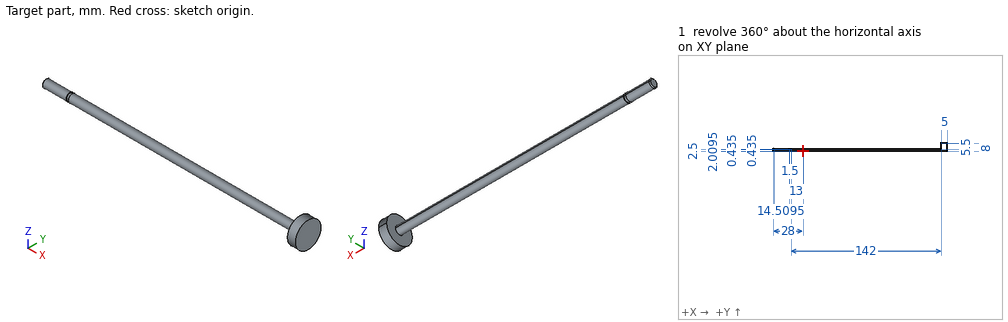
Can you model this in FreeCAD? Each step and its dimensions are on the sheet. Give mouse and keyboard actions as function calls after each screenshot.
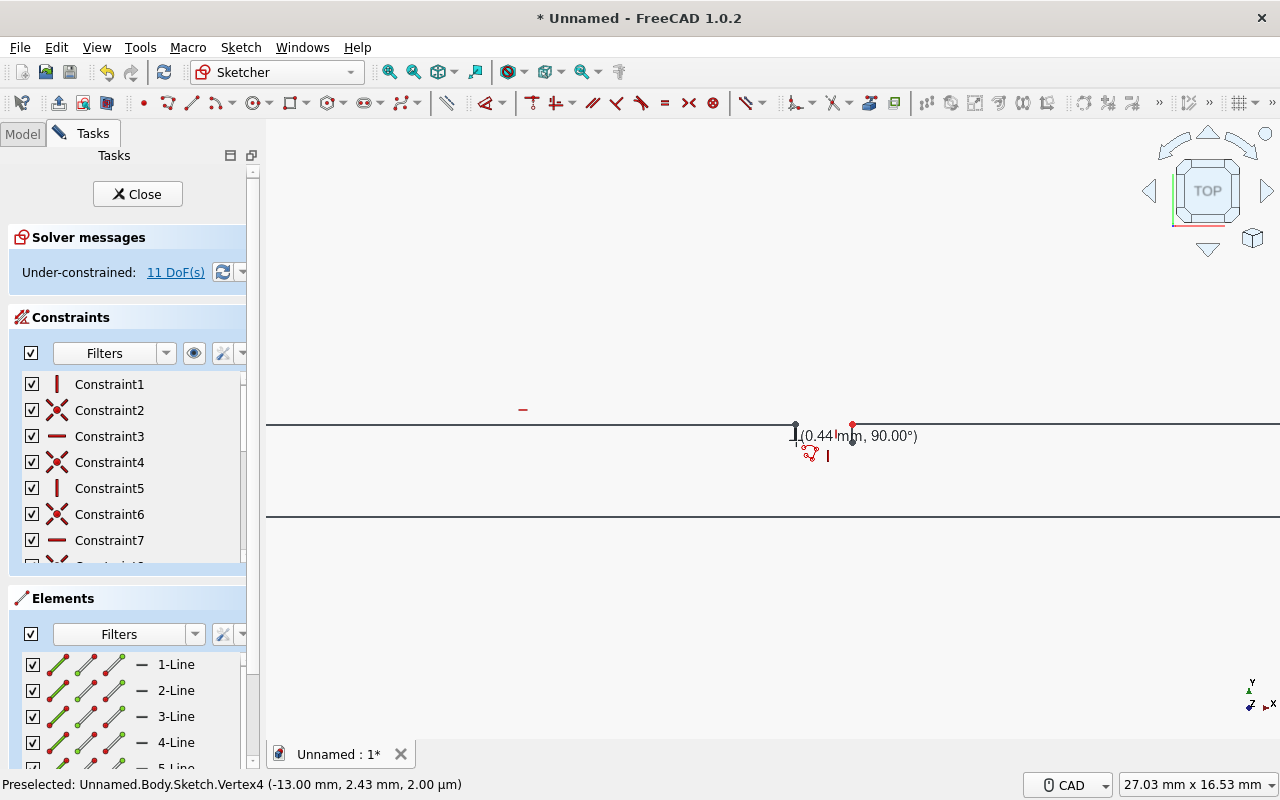
click(796, 440)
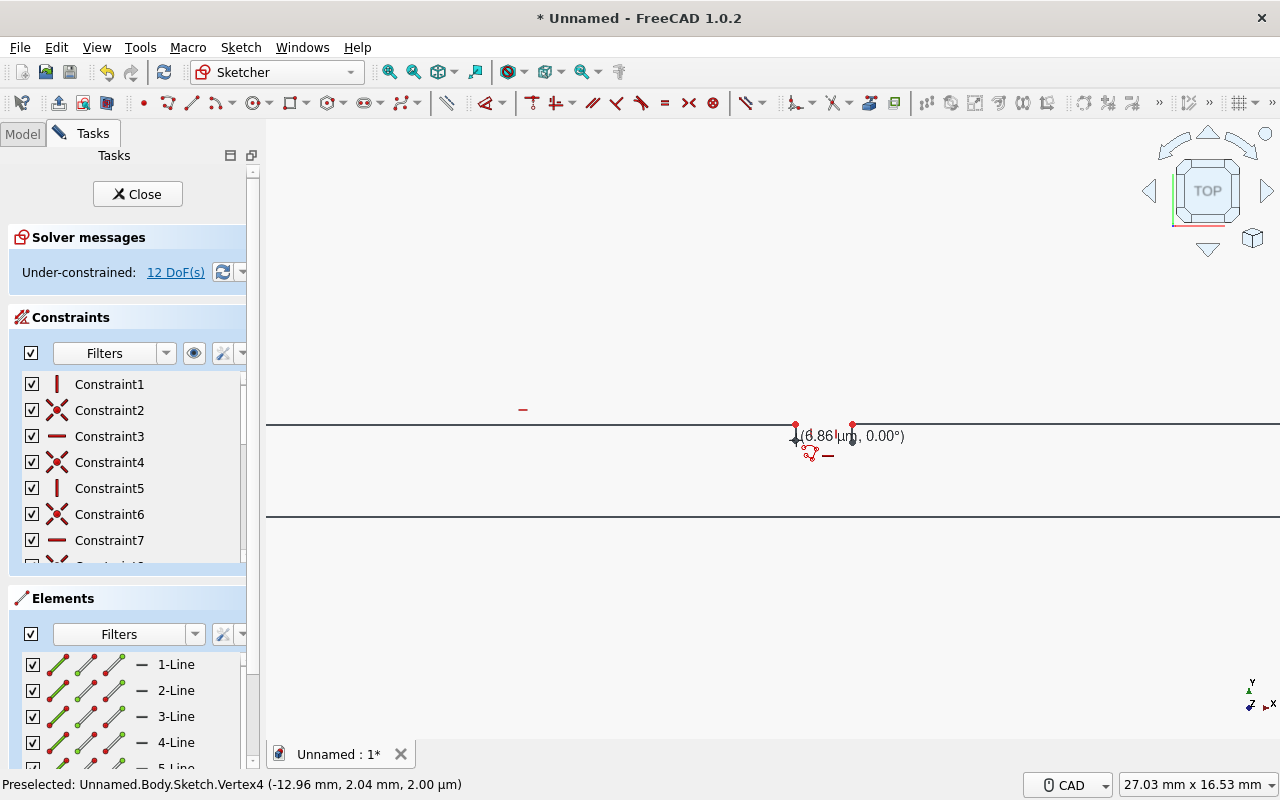
scroll(852, 440, up, 4)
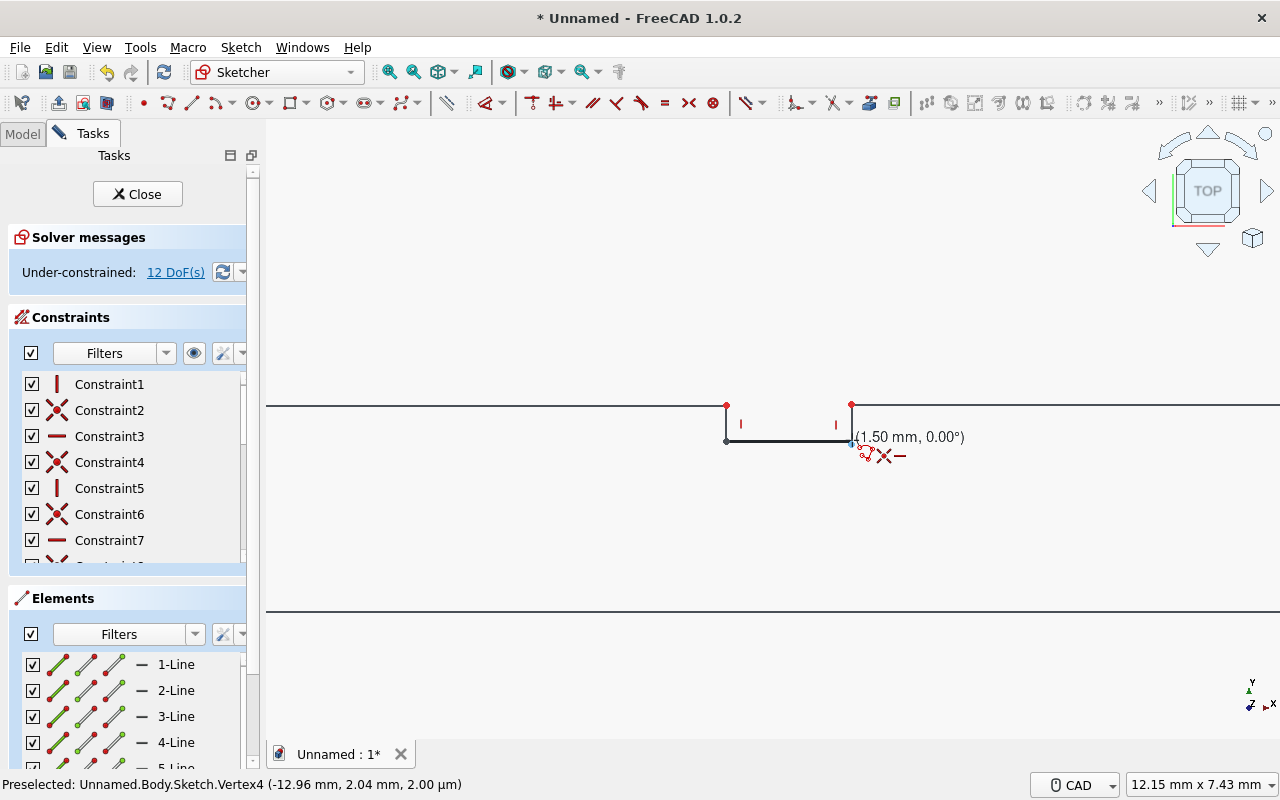
click(852, 435)
key(Escape)
key(Escape)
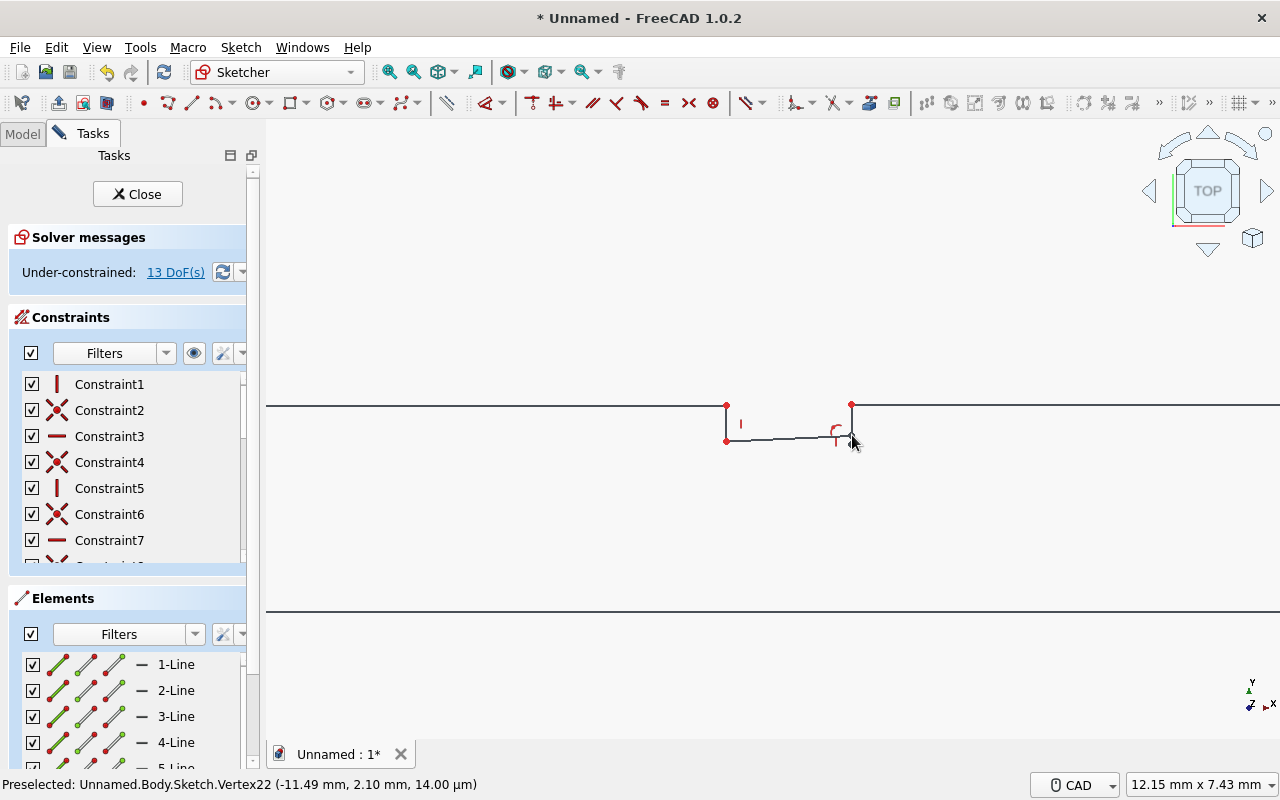
click(764, 440)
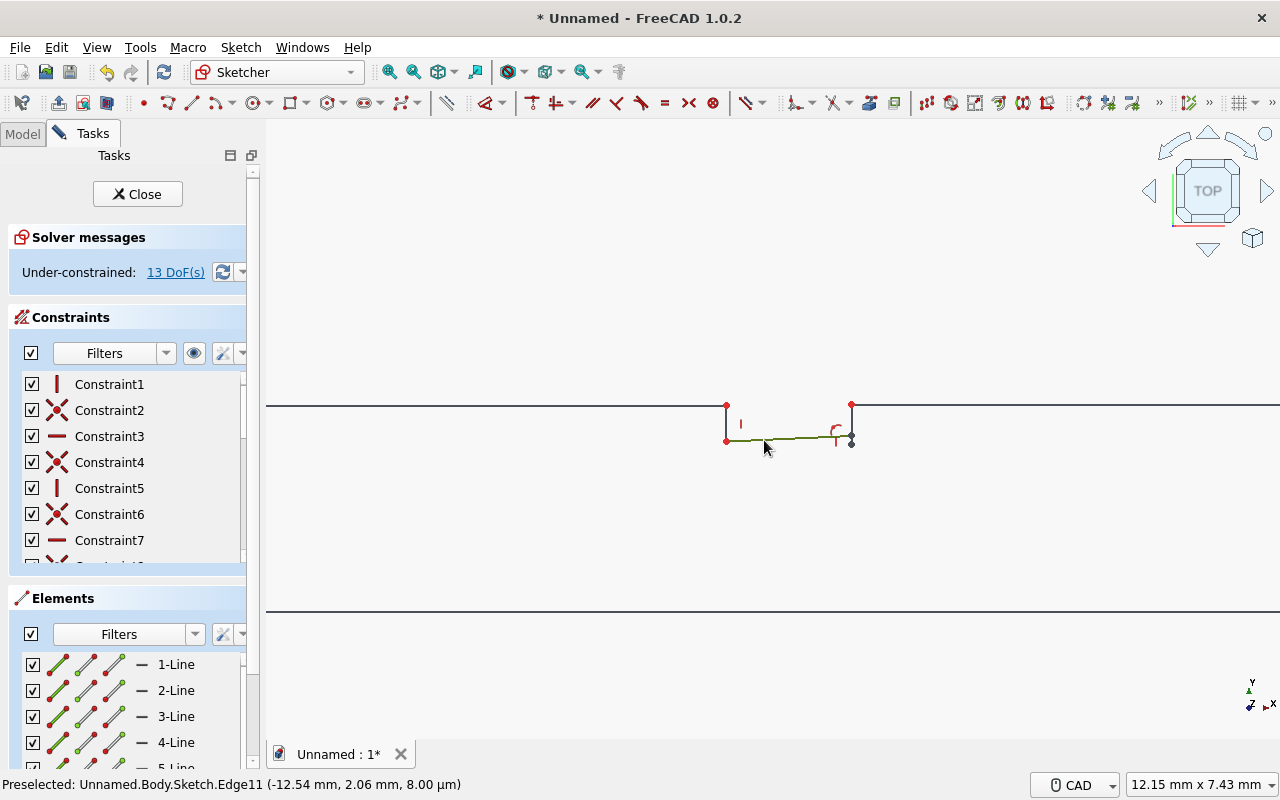
key(h)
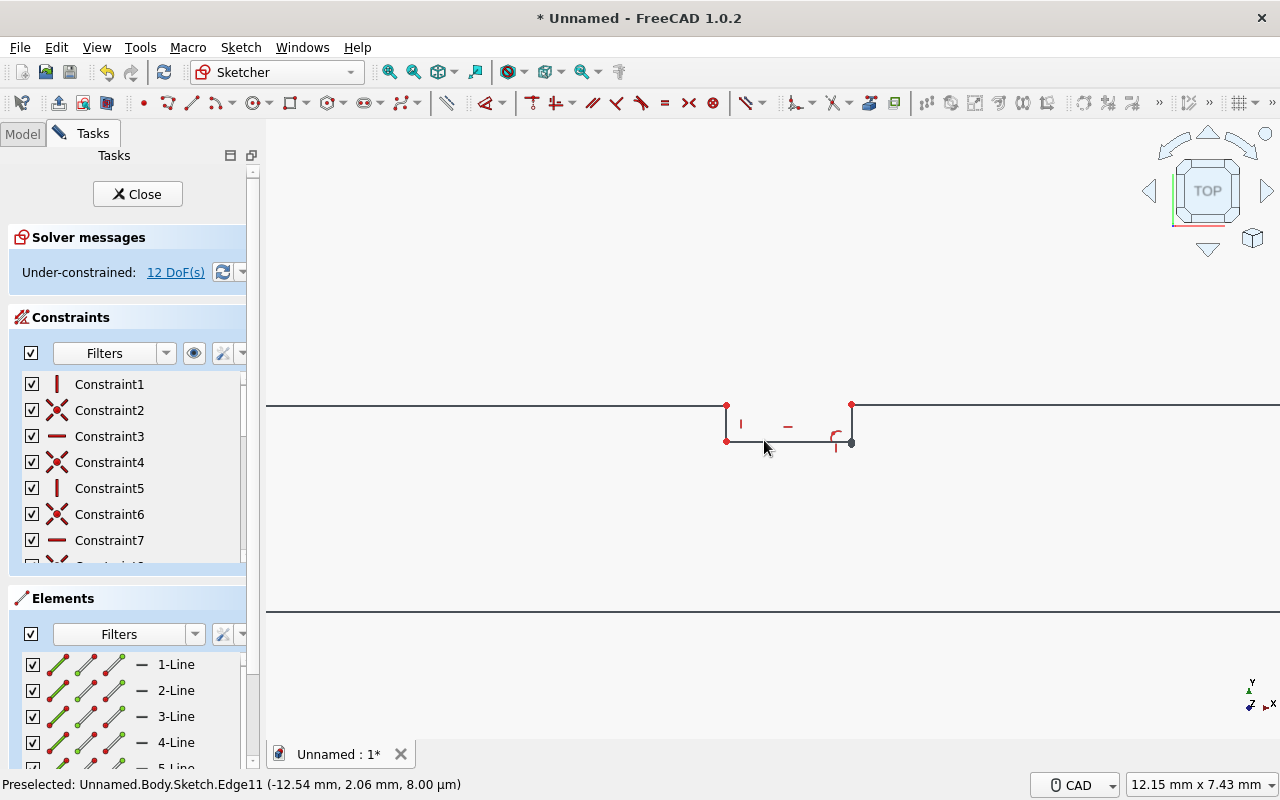
click(486, 104)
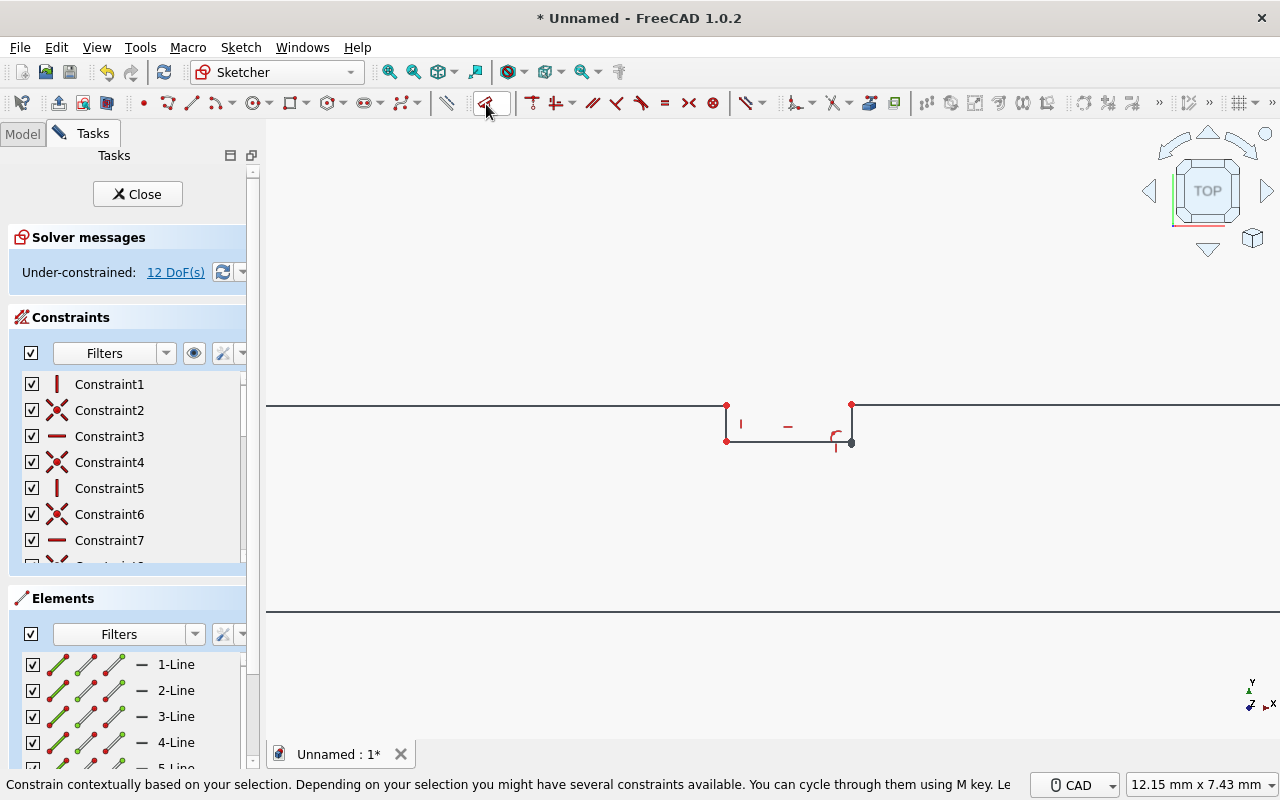
scroll(411, 437, down, 15)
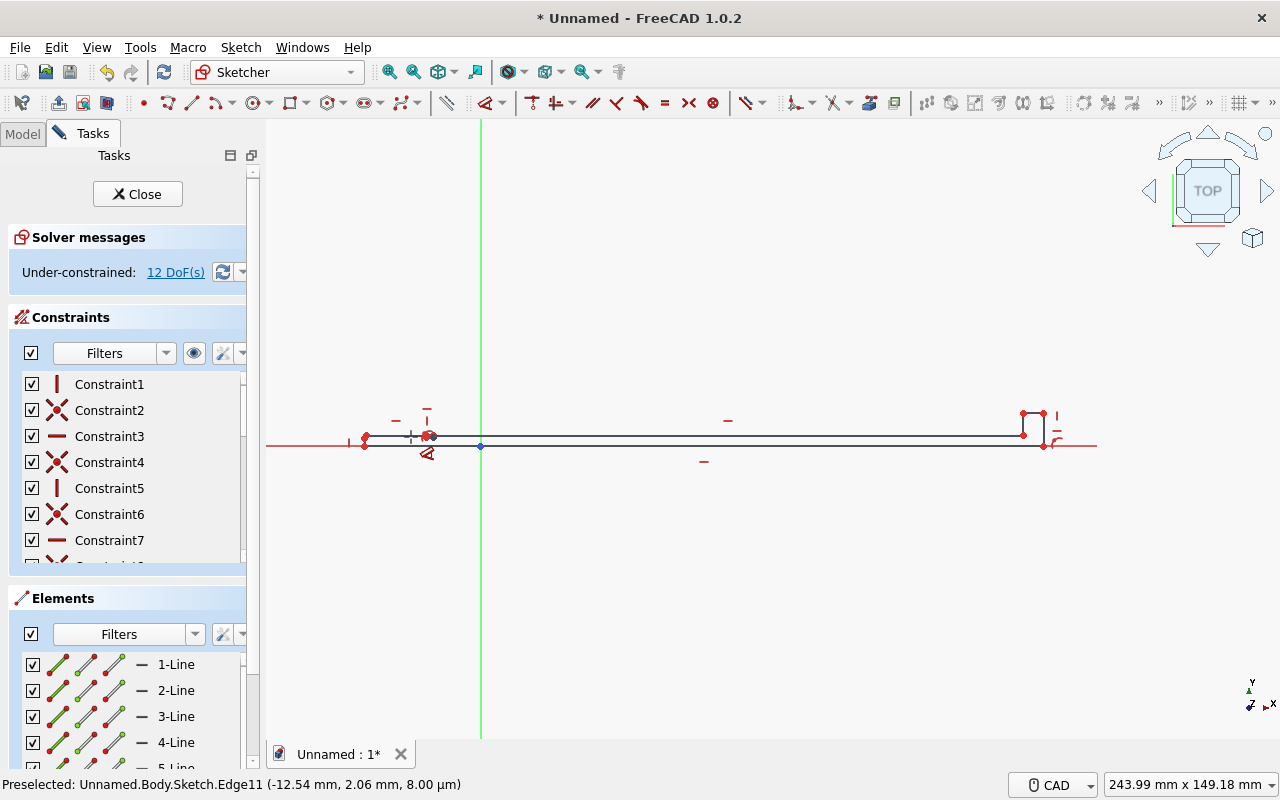
scroll(1030, 413, up, 5)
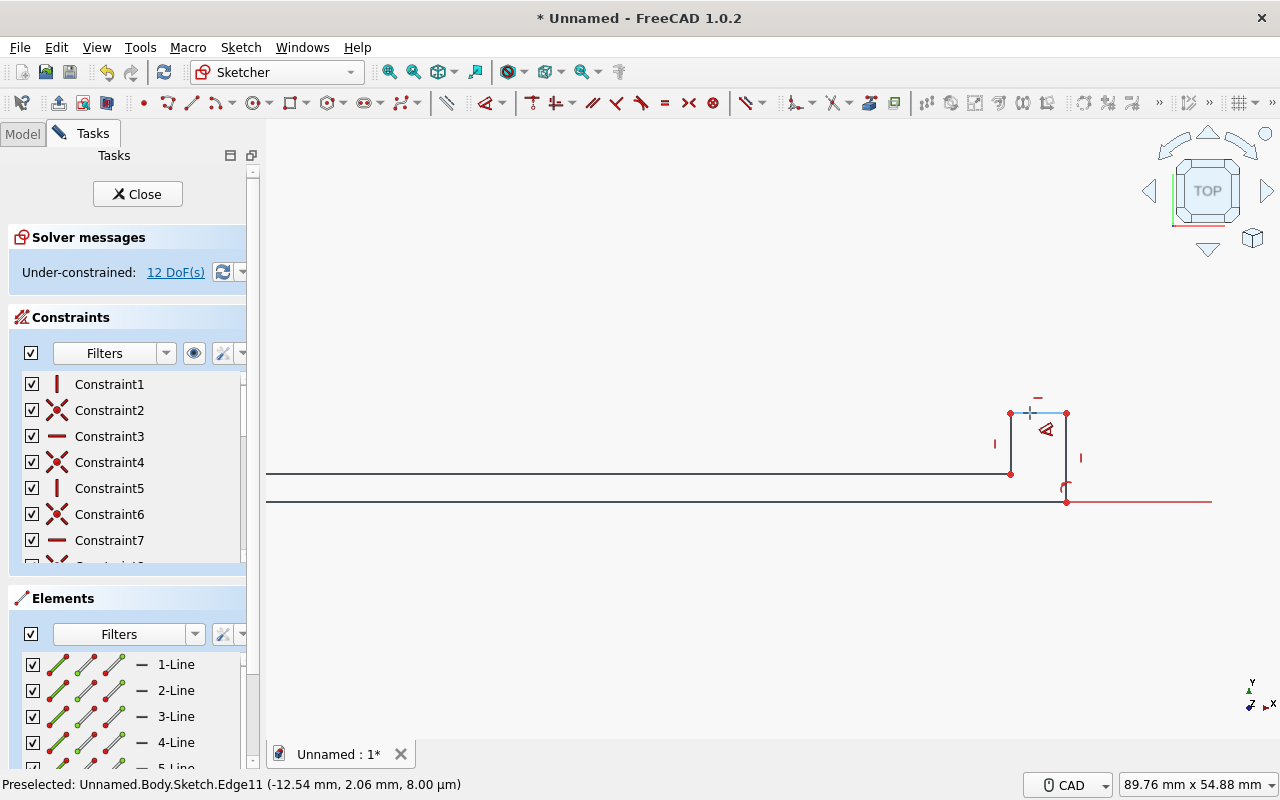
click(1027, 413)
click(1038, 379)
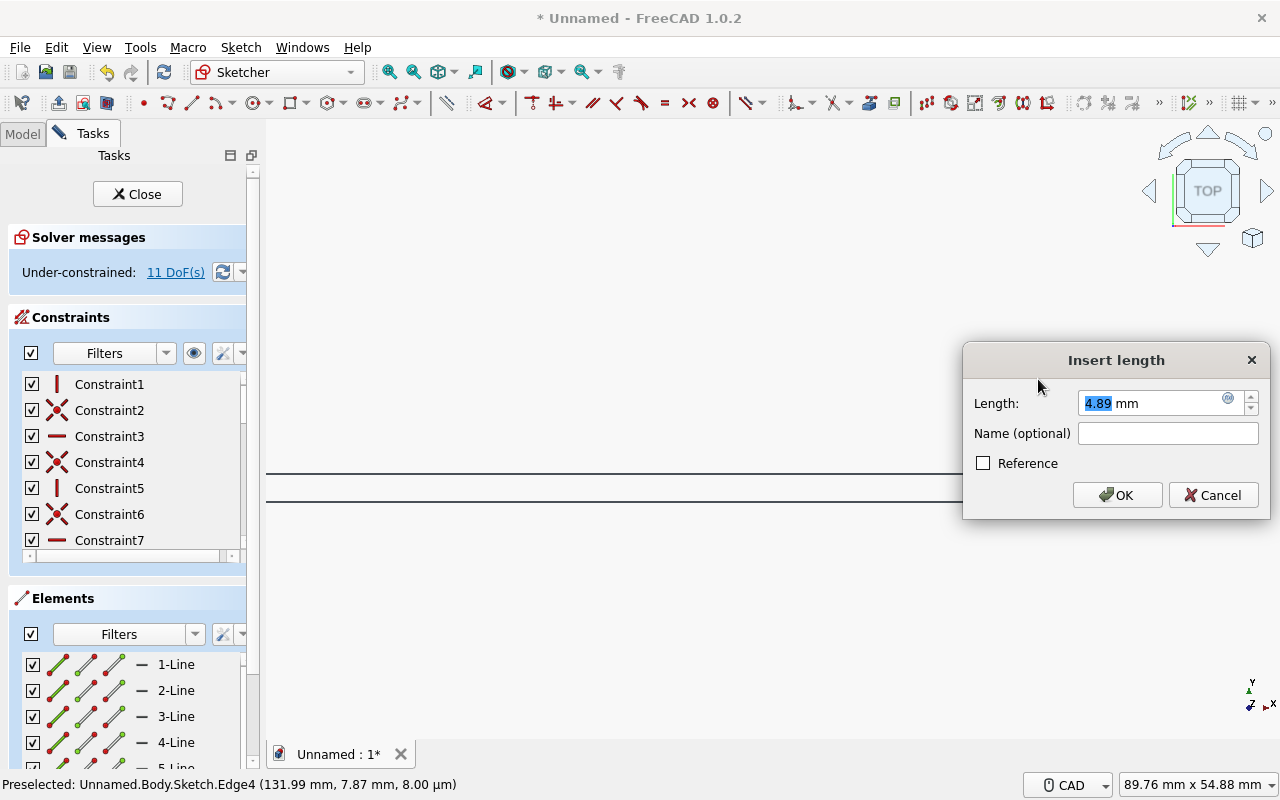
text(5)
key(Return)